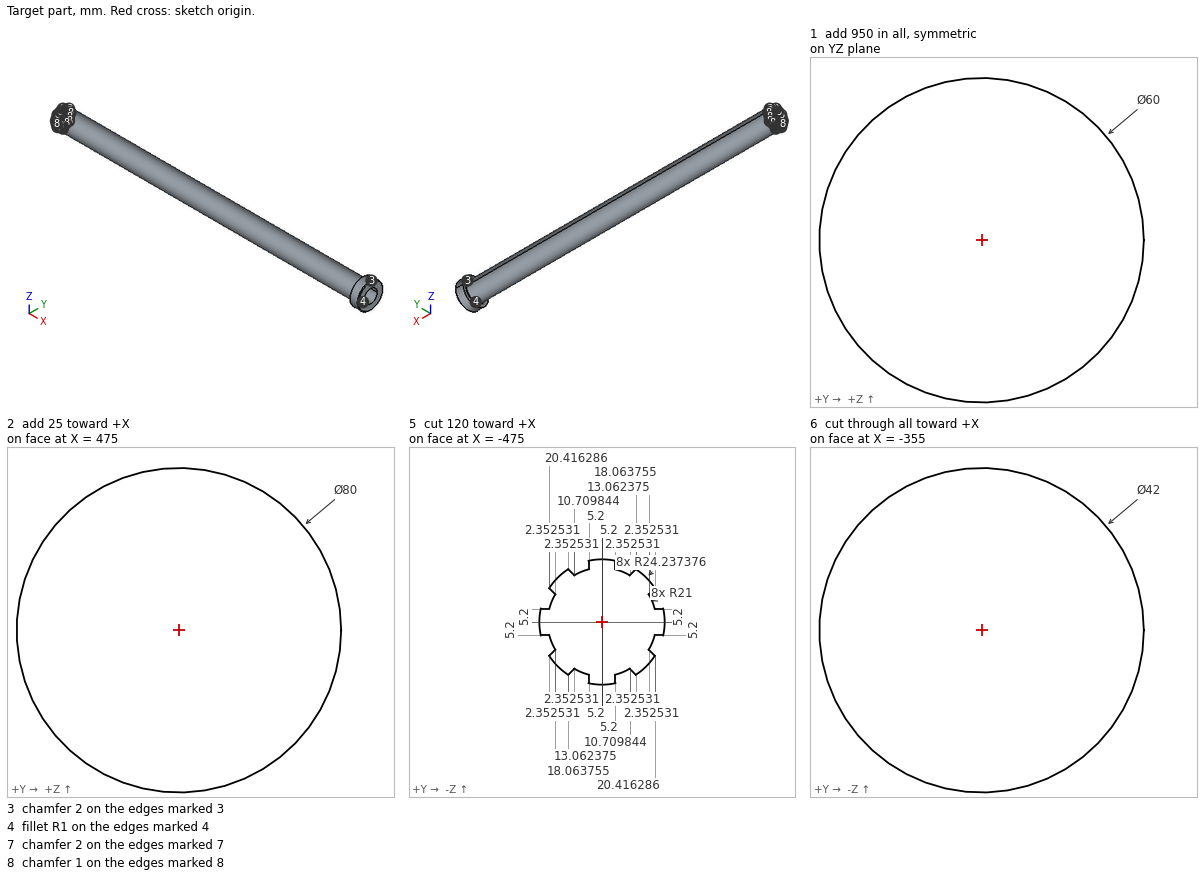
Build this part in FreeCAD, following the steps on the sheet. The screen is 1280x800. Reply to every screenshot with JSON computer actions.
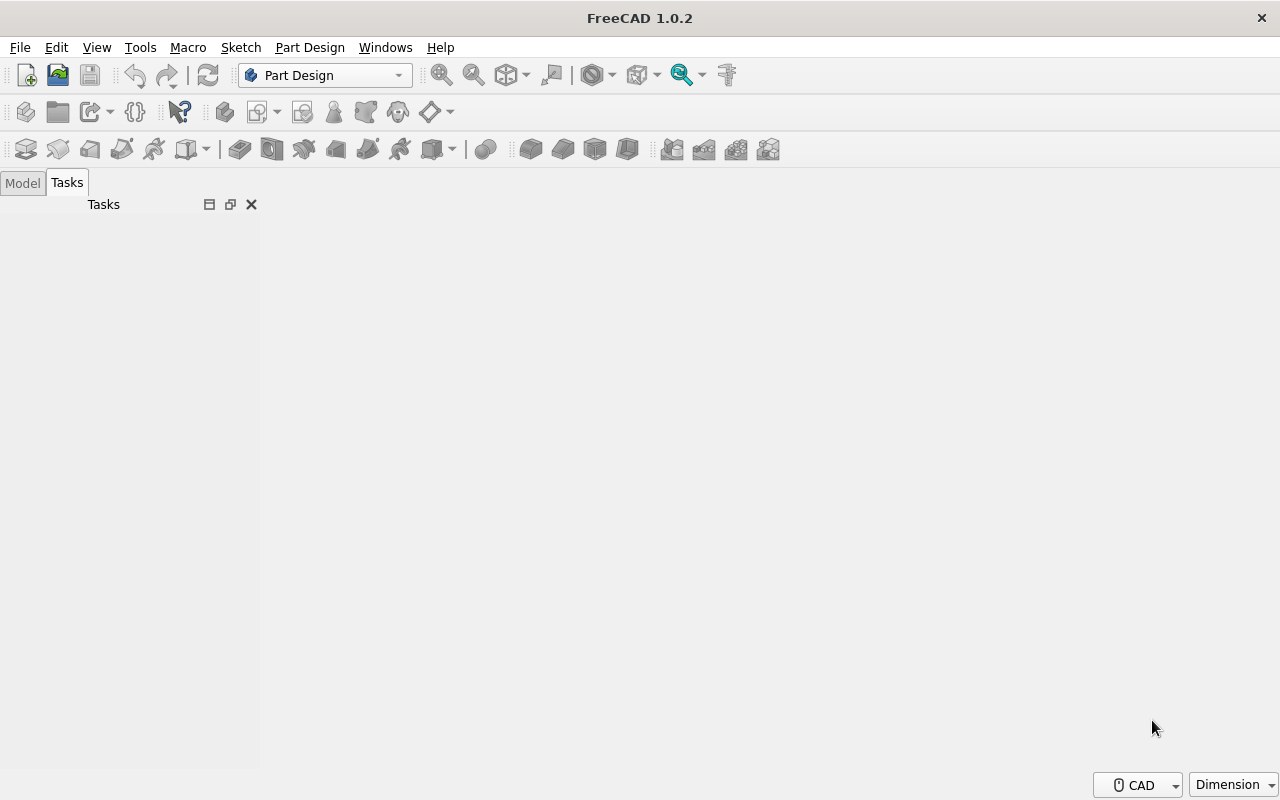
{"action": "key", "text": "ctrl+n"}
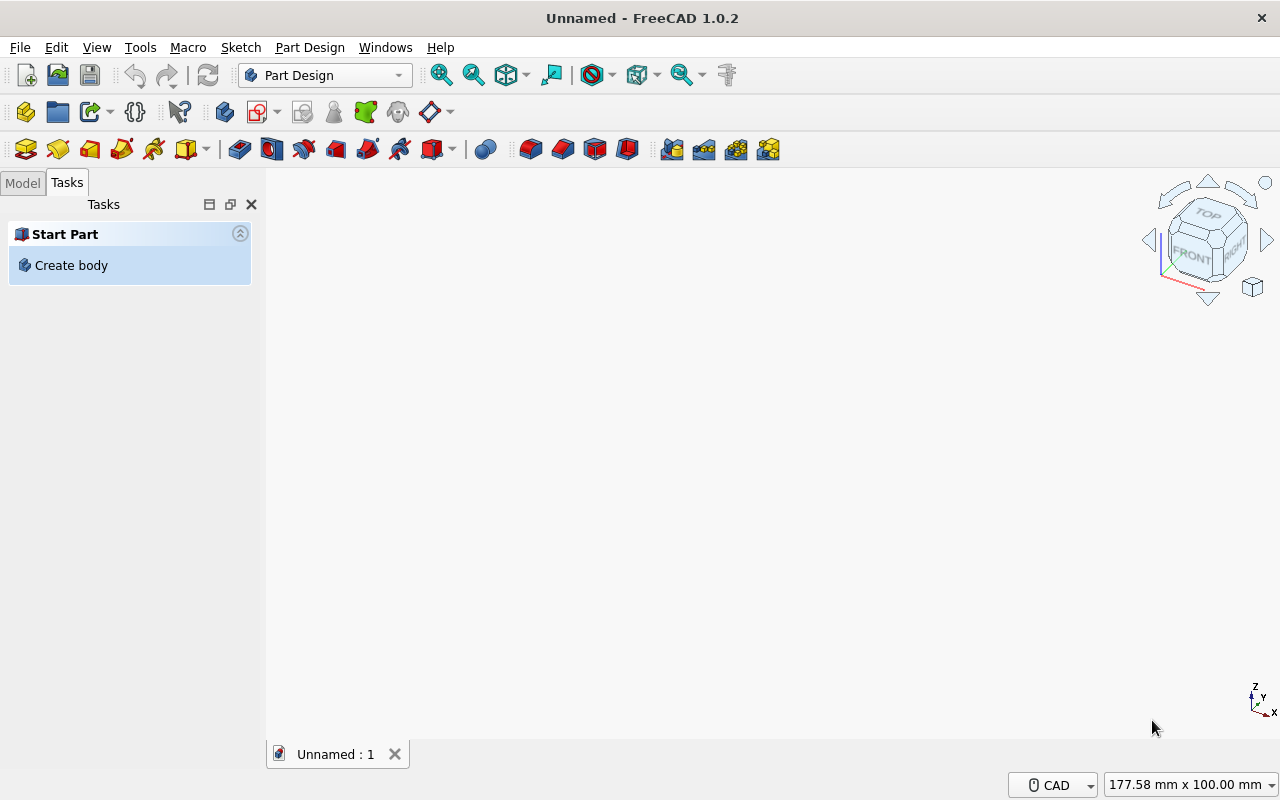
{"action": "left_click", "coordinate": [258, 112]}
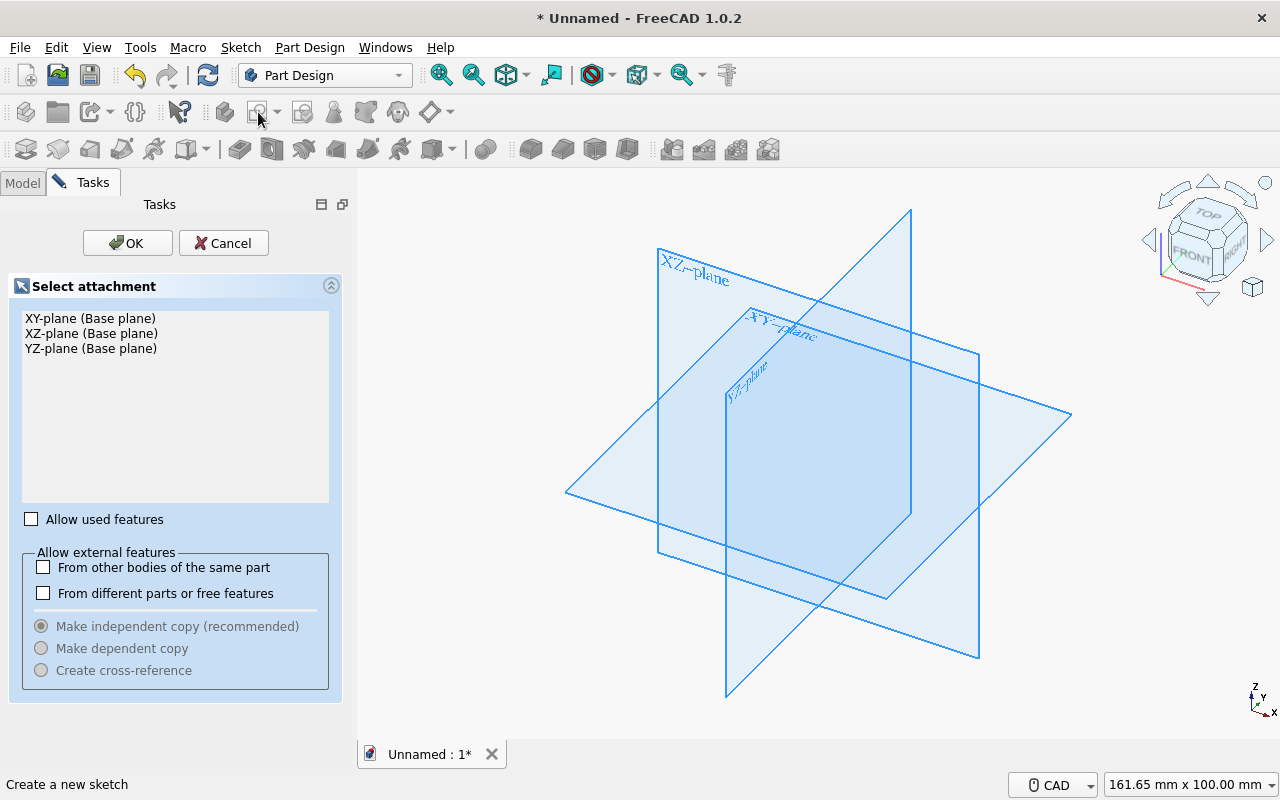
{"action": "left_click", "coordinate": [82, 348]}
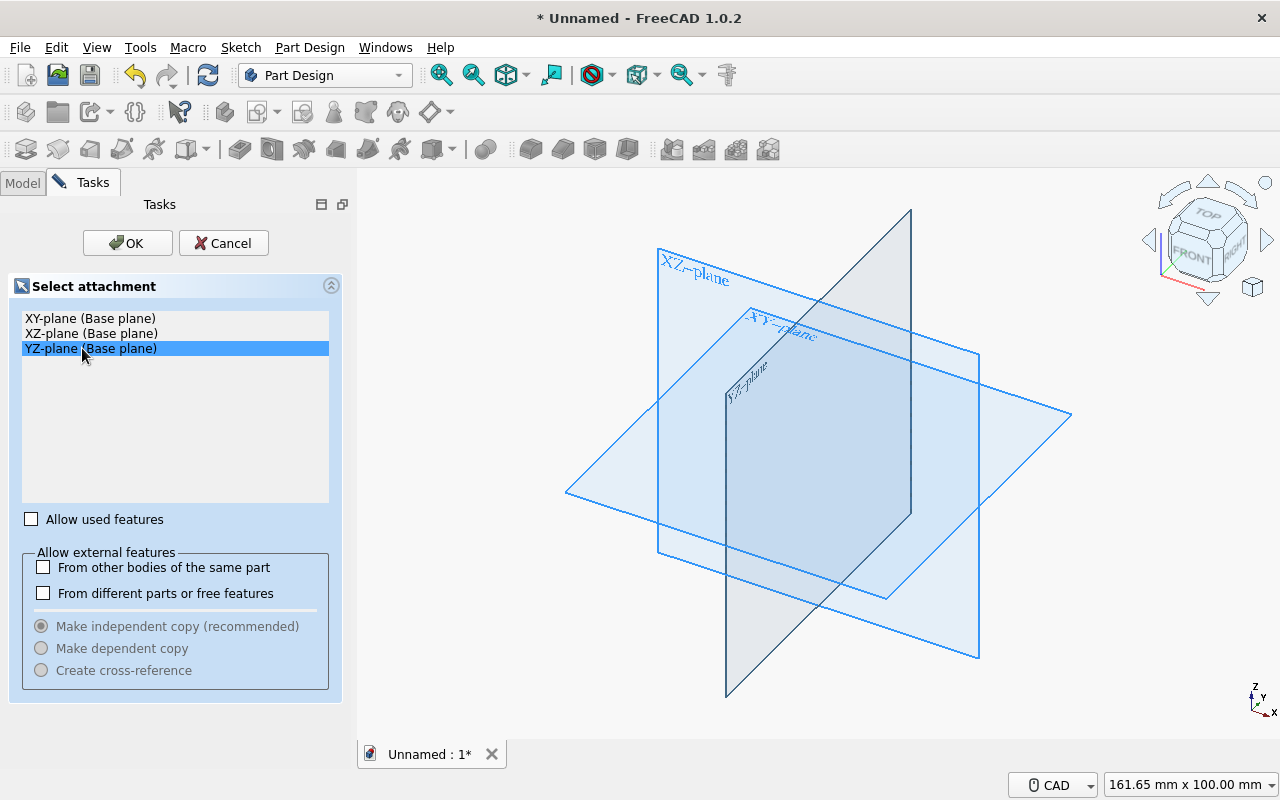
{"action": "left_click", "coordinate": [128, 243]}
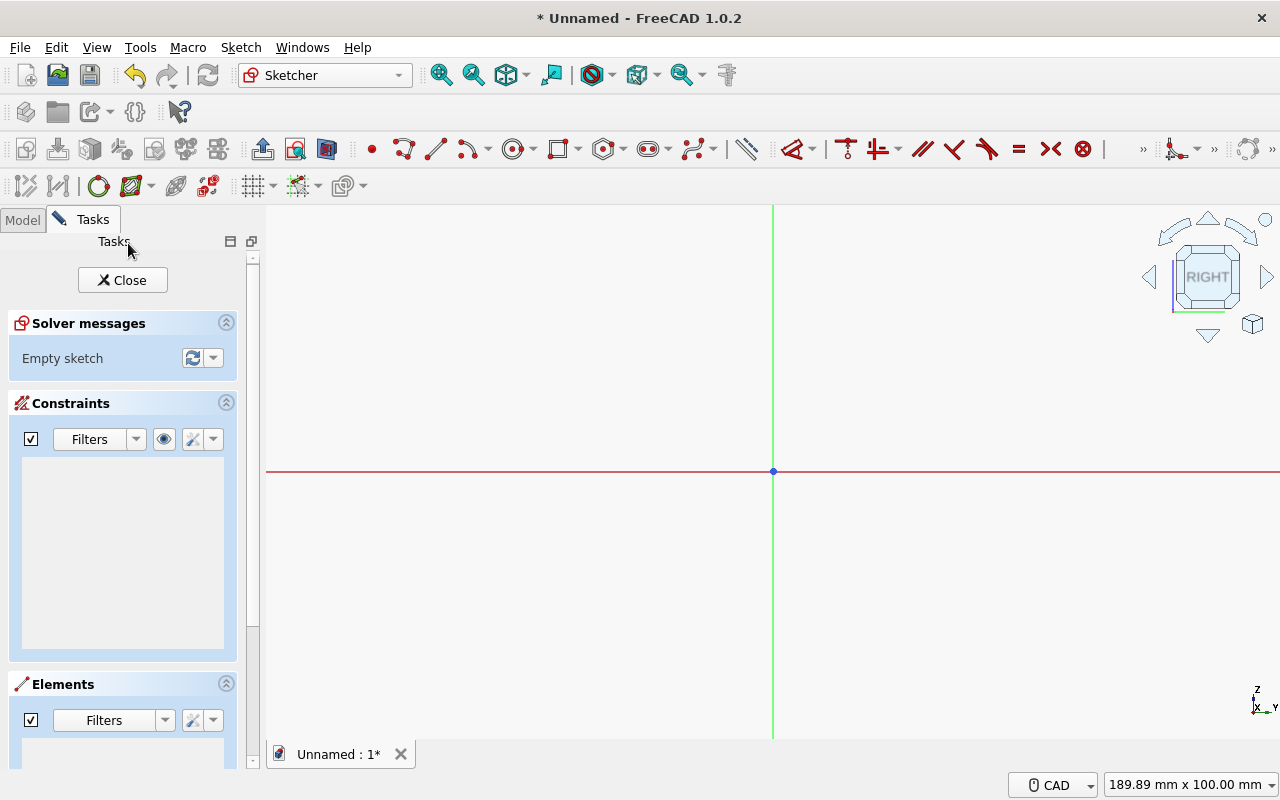
{"action": "key", "text": "g c"}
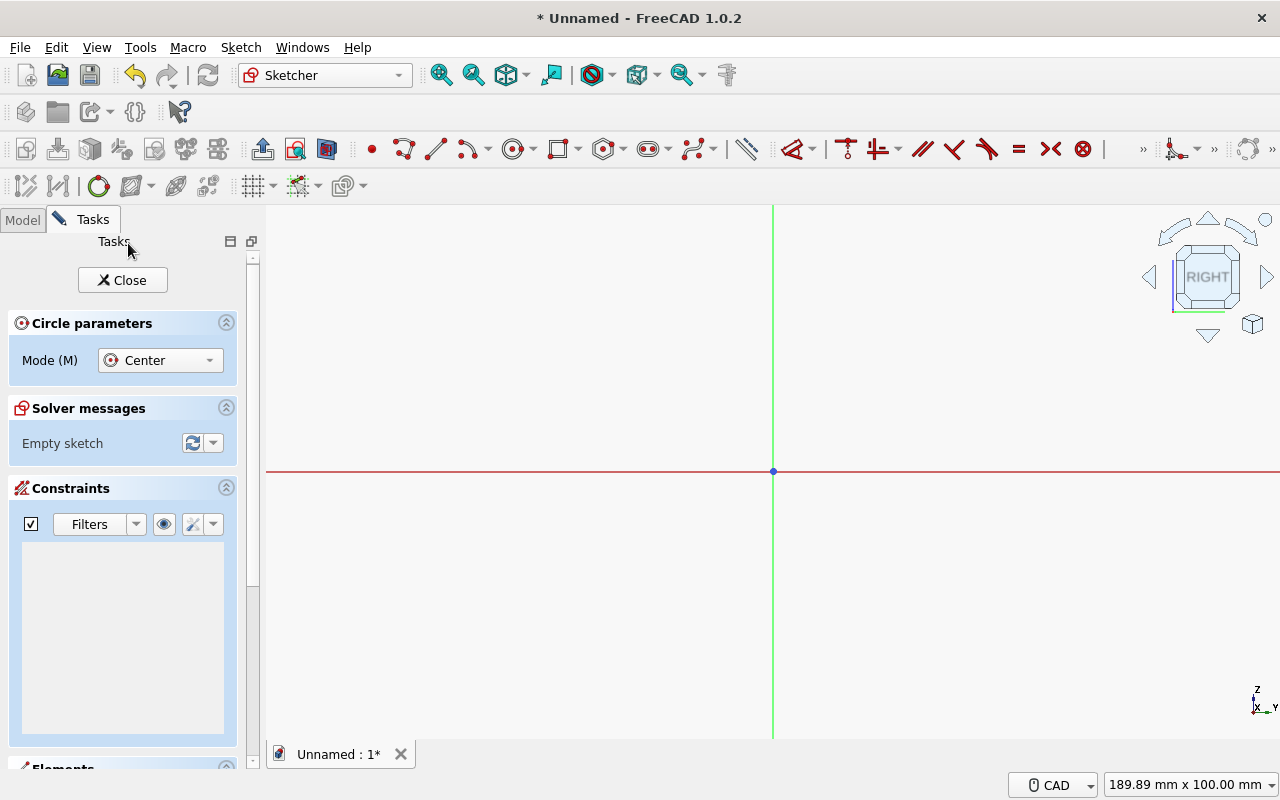
{"action": "left_click", "coordinate": [773, 472]}
{"action": "mouse_move", "coordinate": [886, 359]}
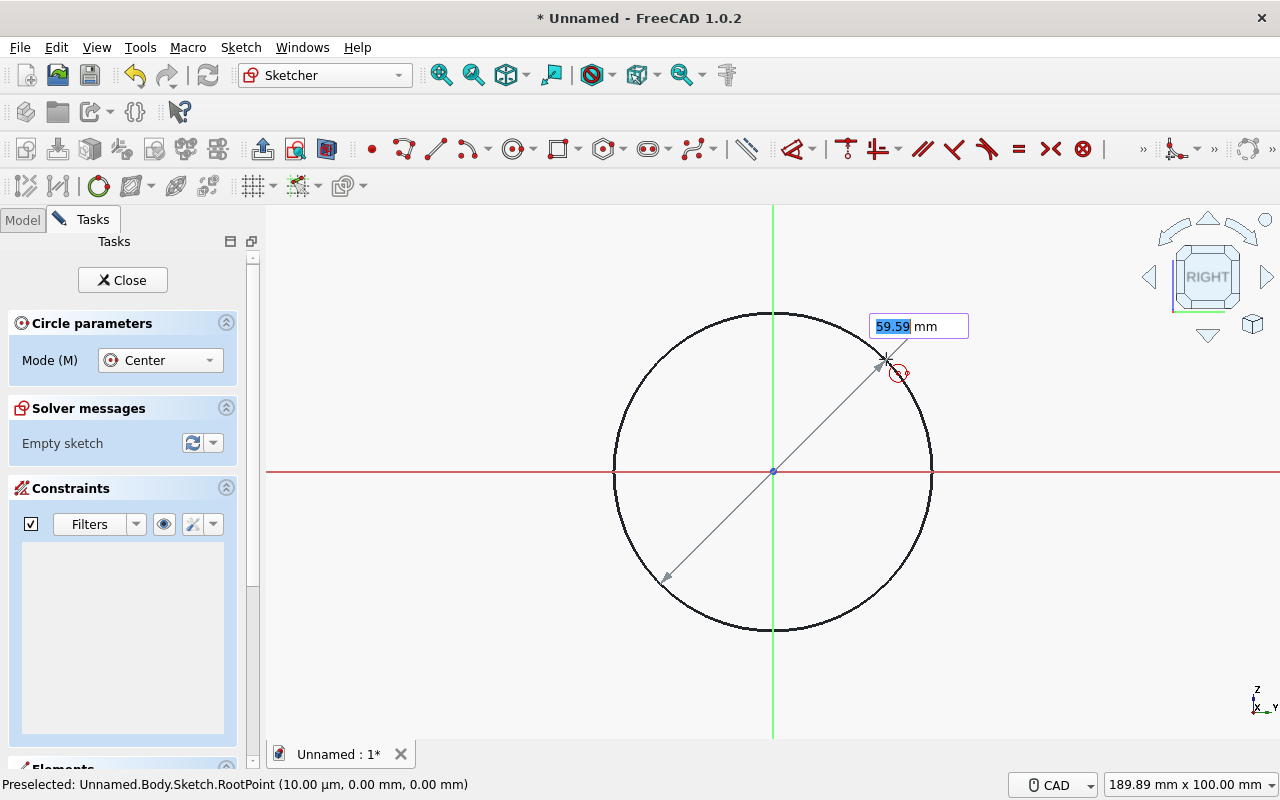
{"action": "type", "text": "60"}
{"action": "key", "text": "Return"}
{"action": "key", "text": "Escape"}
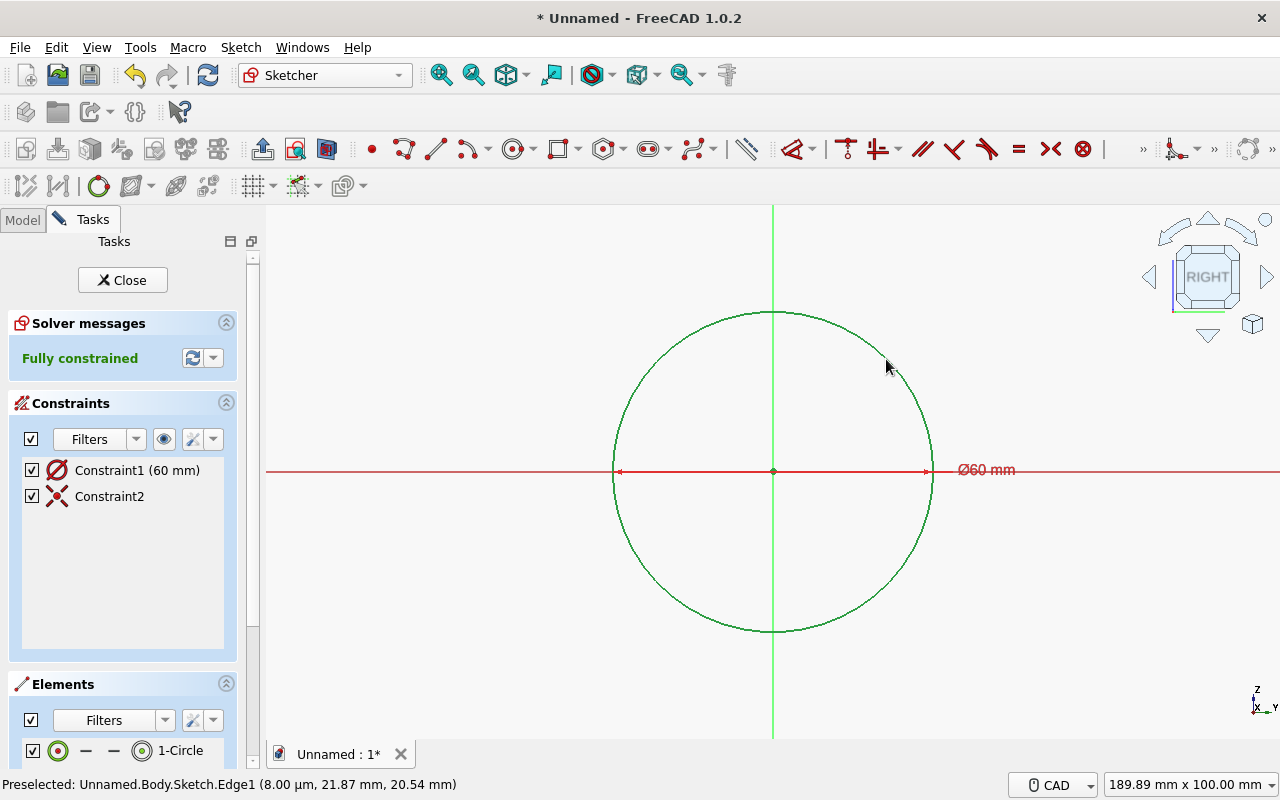
{"action": "left_click", "coordinate": [123, 280]}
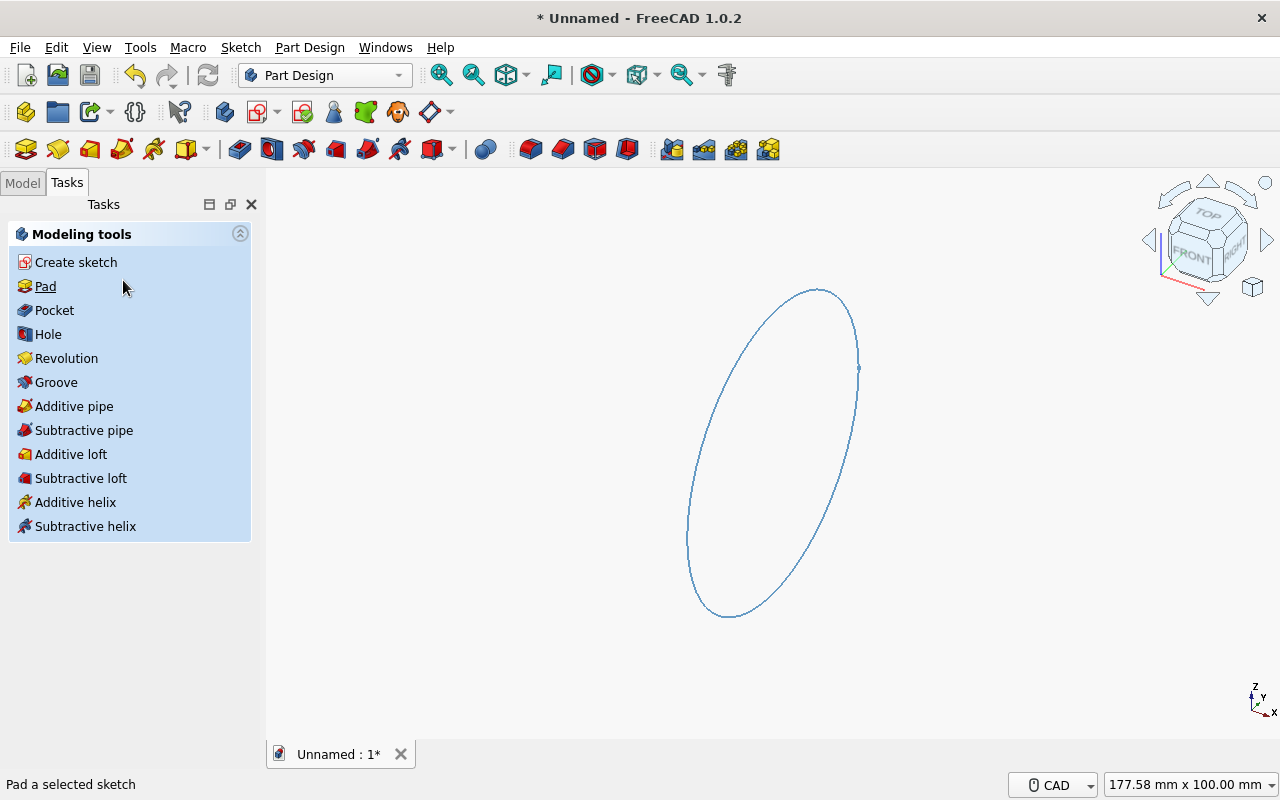
{"action": "left_click", "coordinate": [26, 150]}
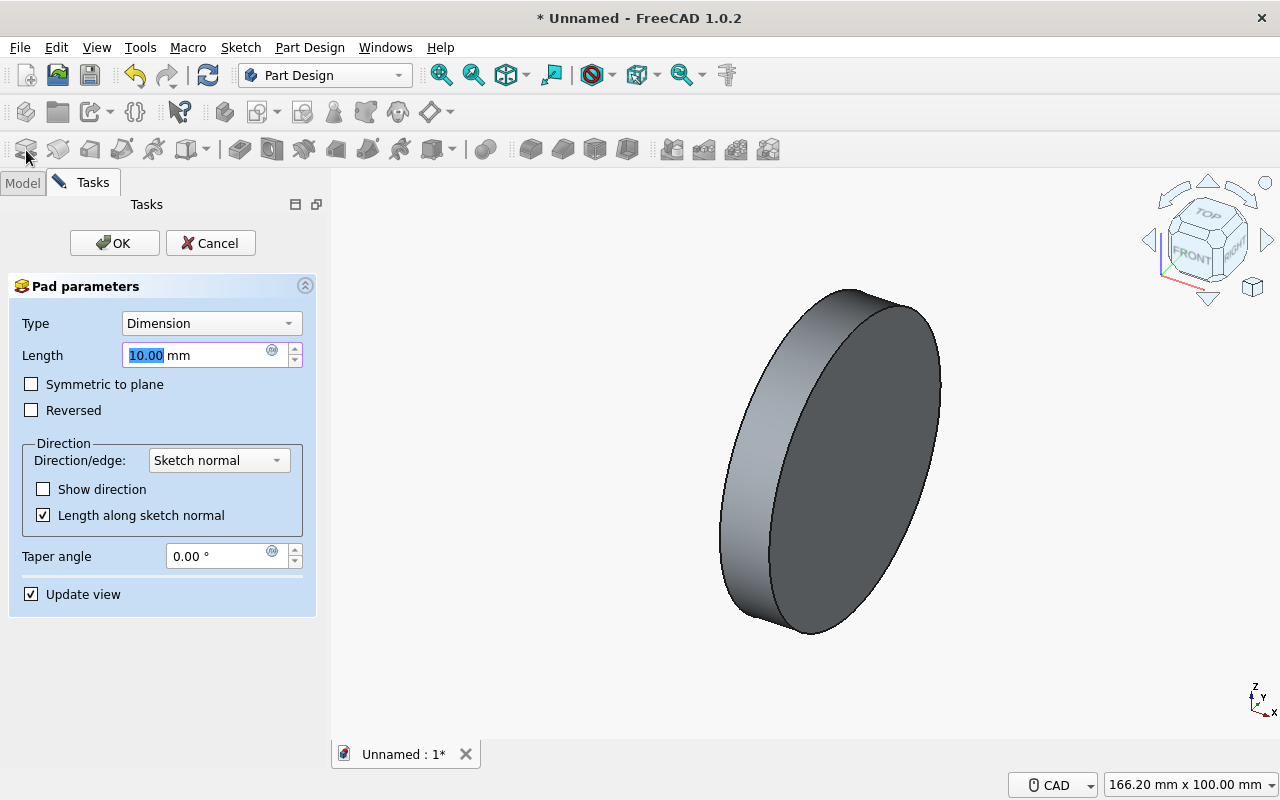
{"action": "type", "text": "950"}
{"action": "key", "text": "Tab"}